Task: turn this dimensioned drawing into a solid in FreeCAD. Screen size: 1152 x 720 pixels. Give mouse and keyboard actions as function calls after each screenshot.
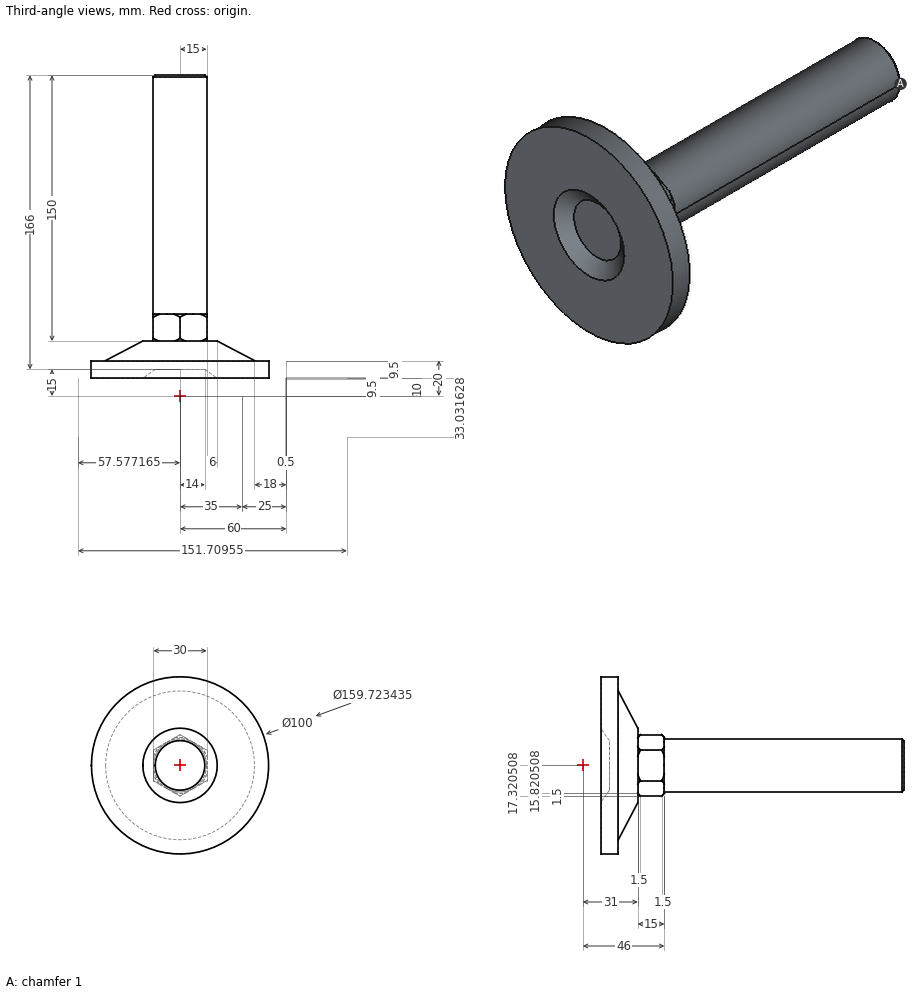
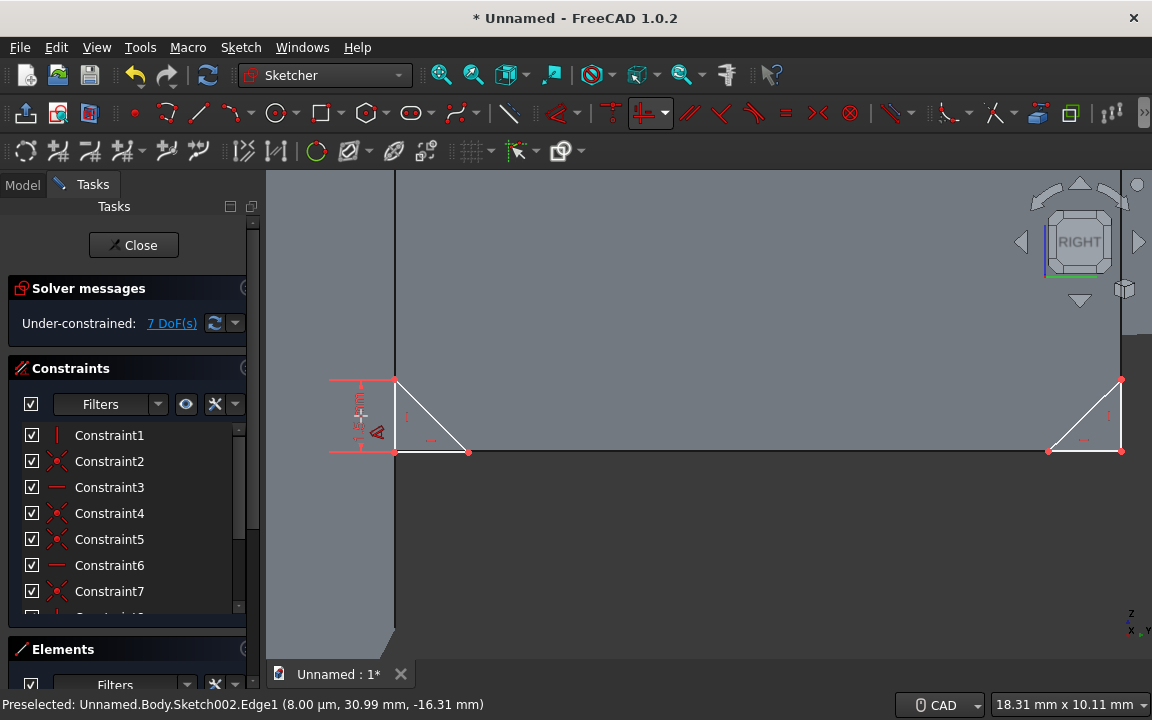
click(417, 452)
click(431, 486)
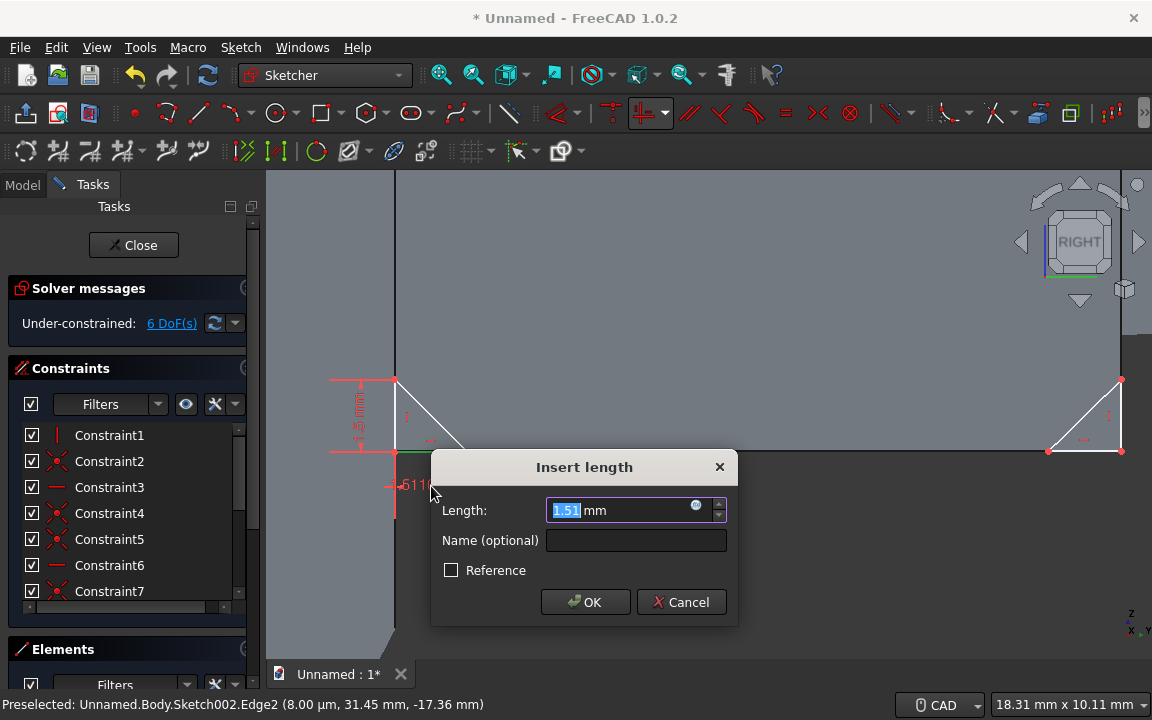
text(1.5)
key(Return)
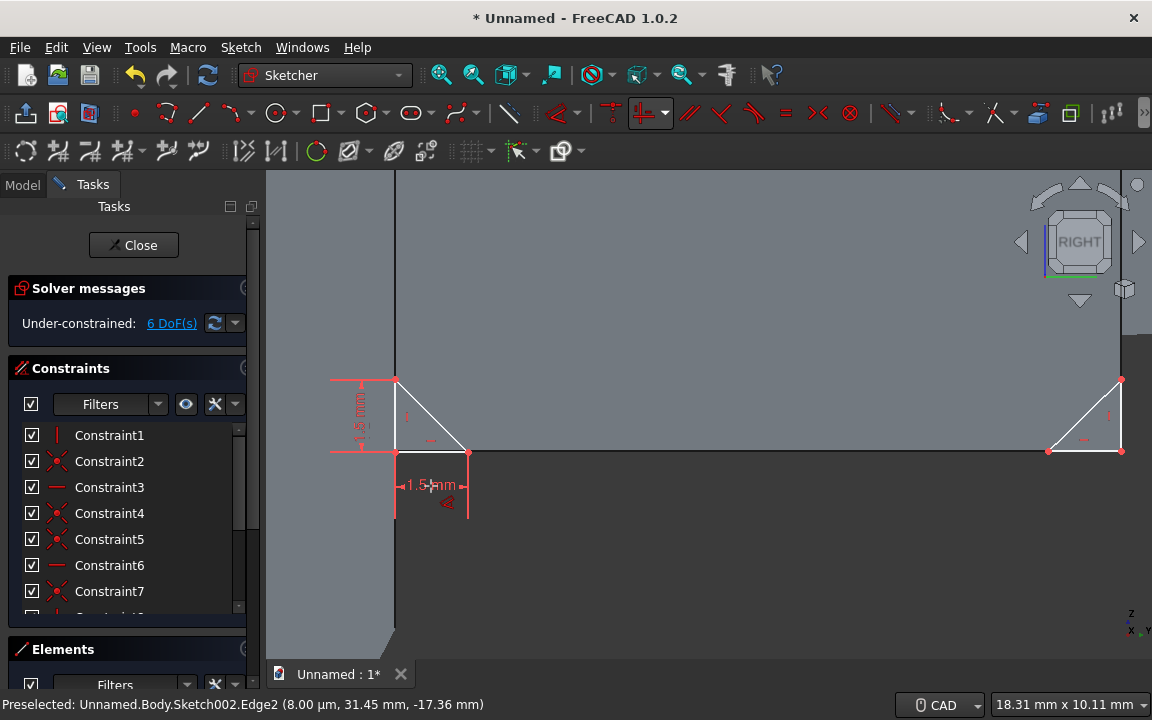
scroll(401, 415, down, 2)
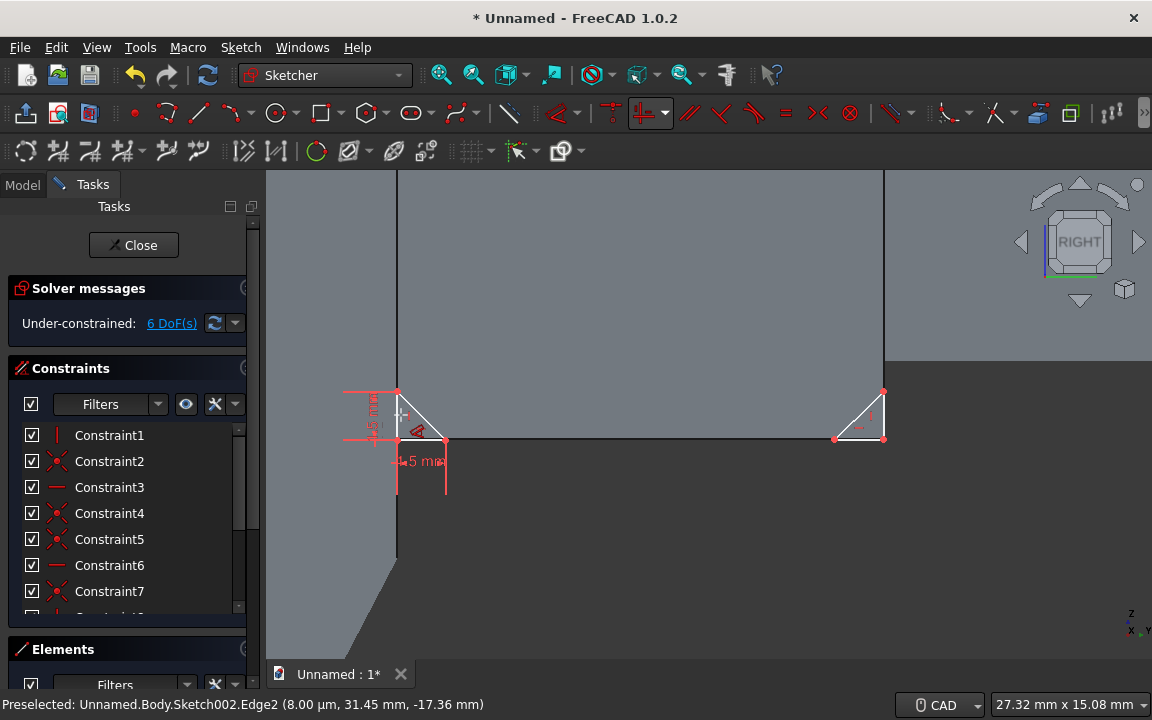
scroll(850, 440, up, 2)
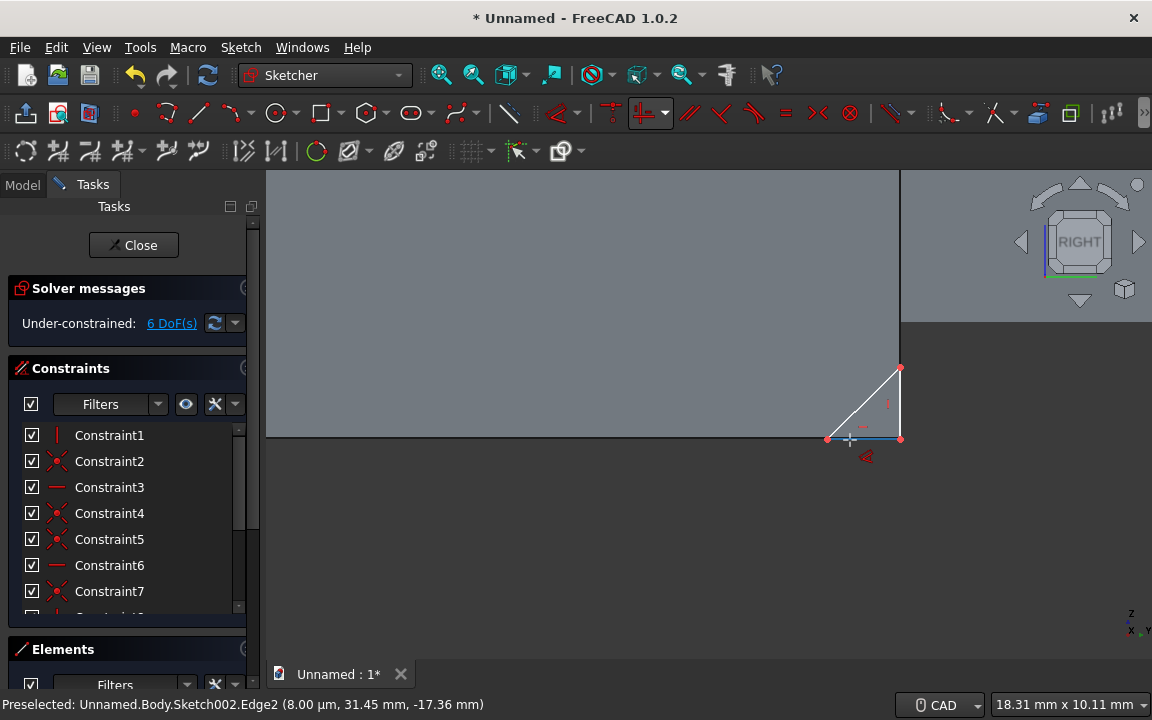
click(849, 439)
click(864, 473)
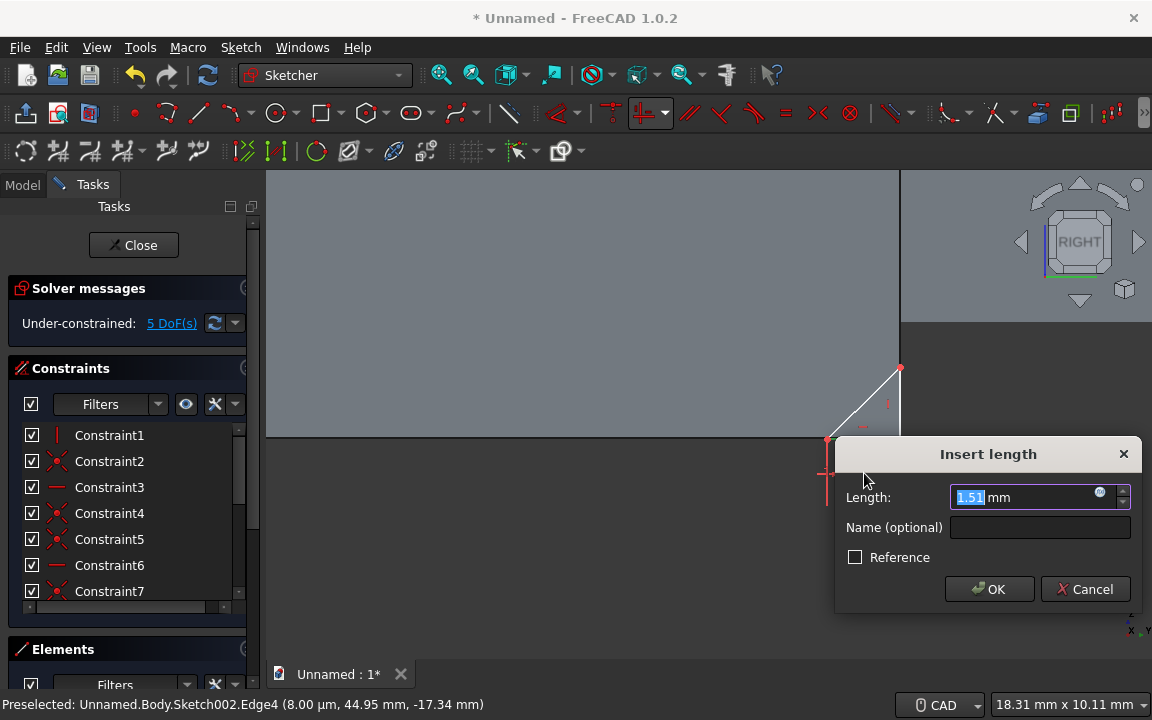
text(1.5)
key(Return)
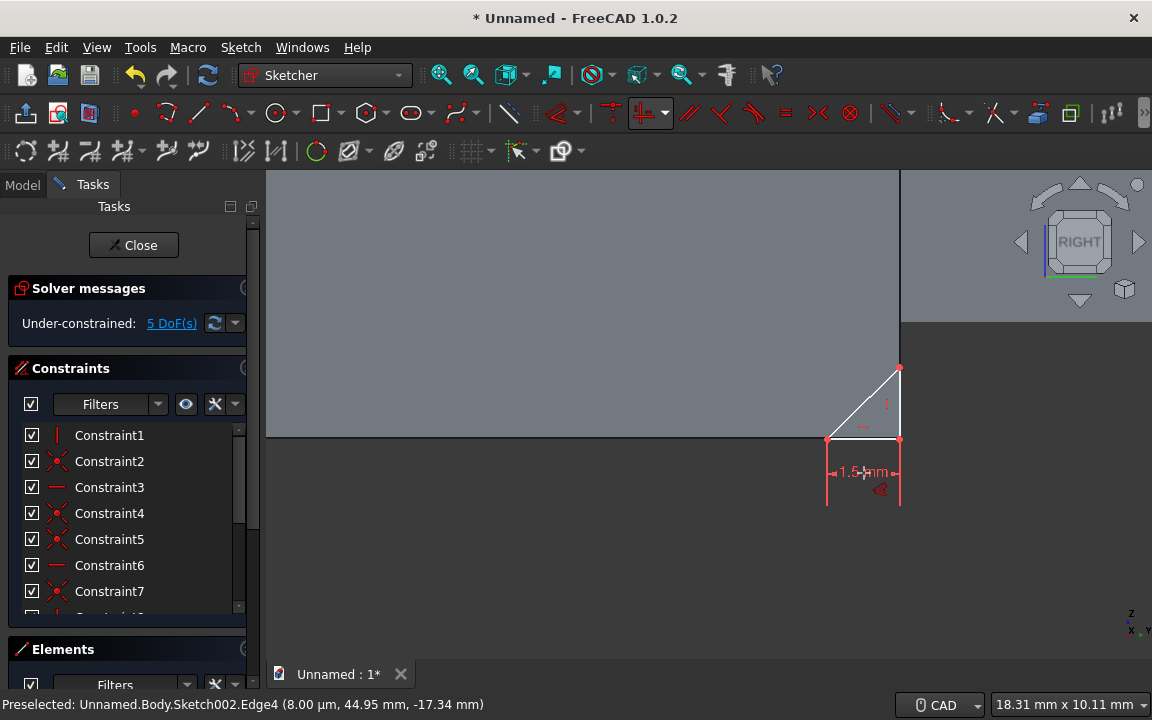
click(900, 418)
click(934, 403)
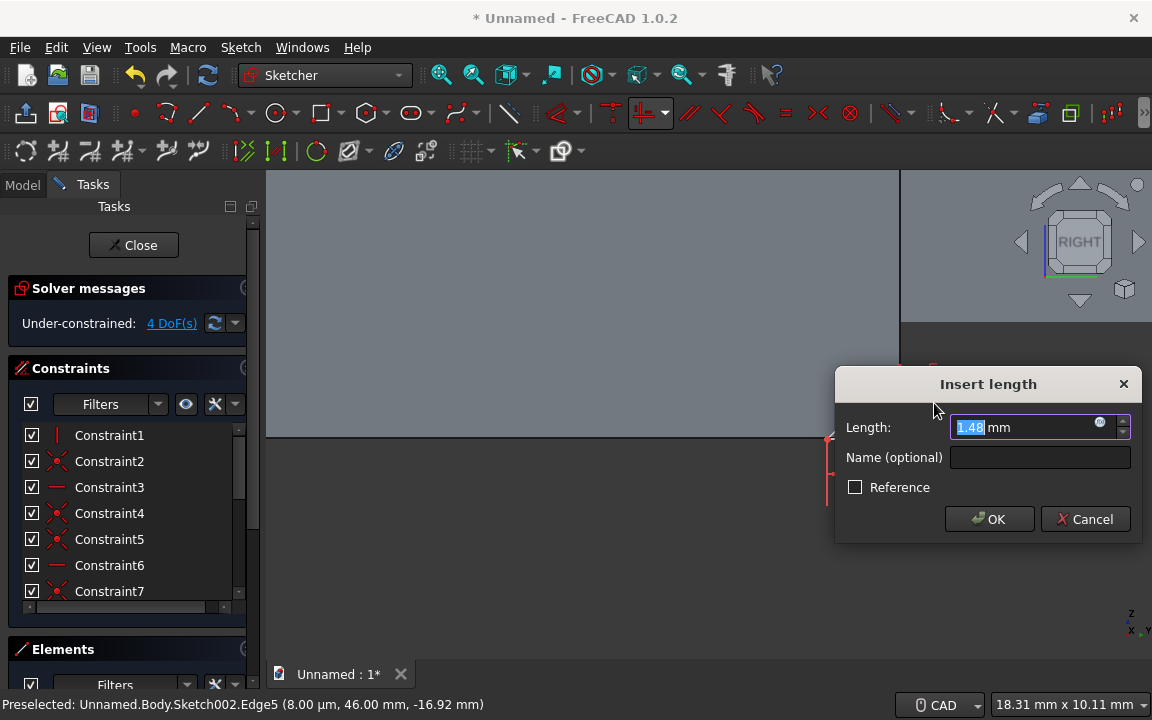
text(1.5)
key(Return)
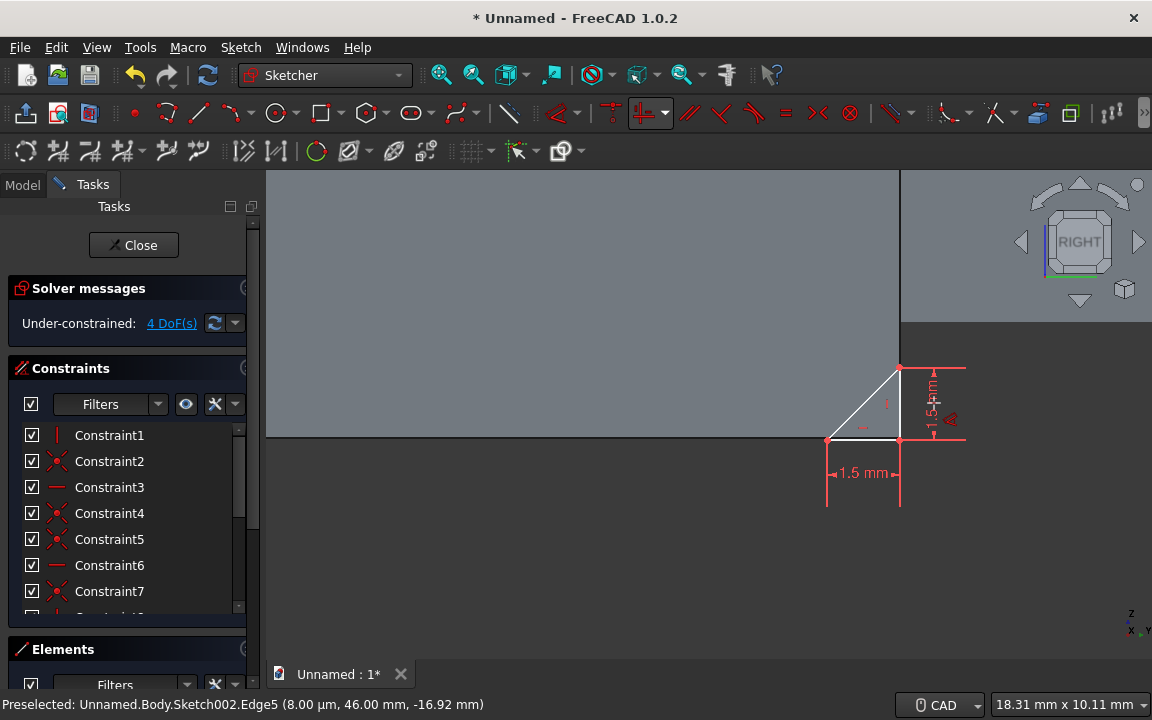
scroll(851, 440, down, 2)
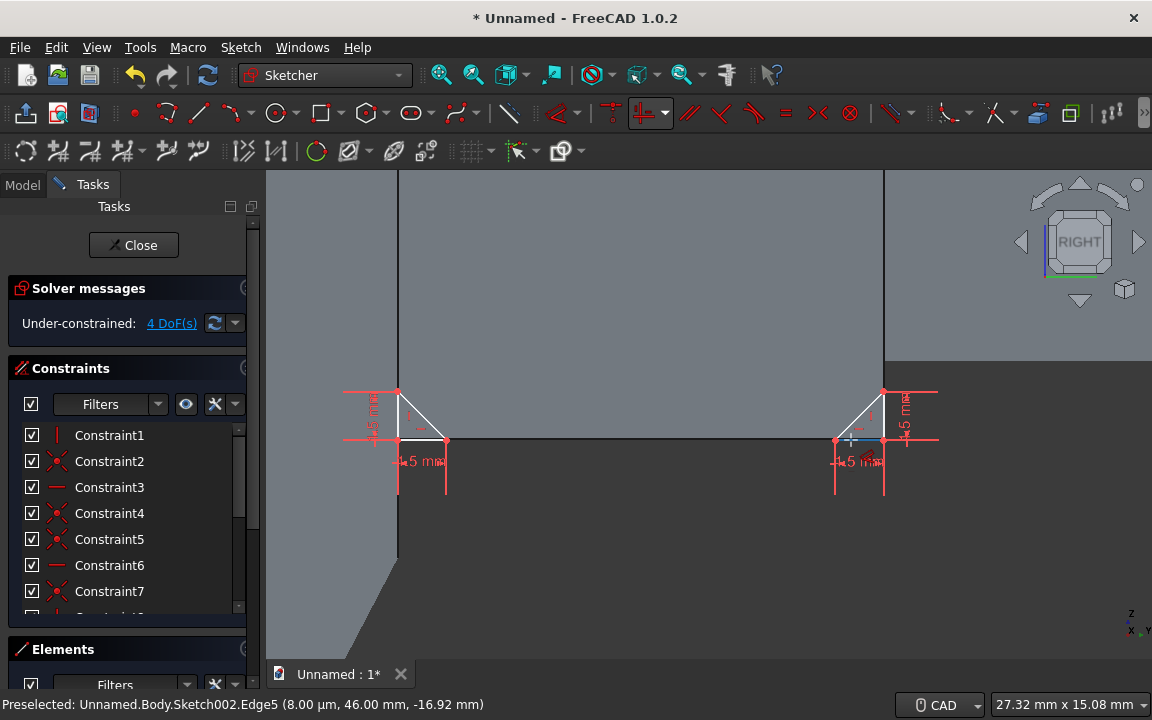
click(398, 392)
click(346, 450)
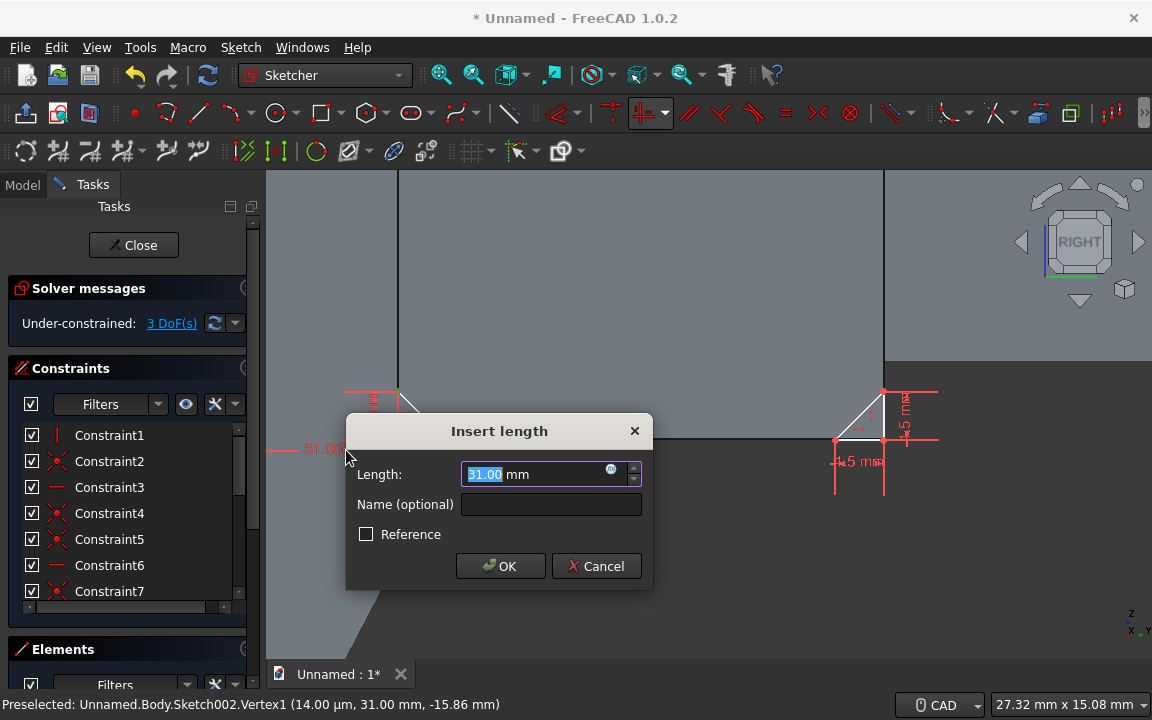
text(31)
key(Return)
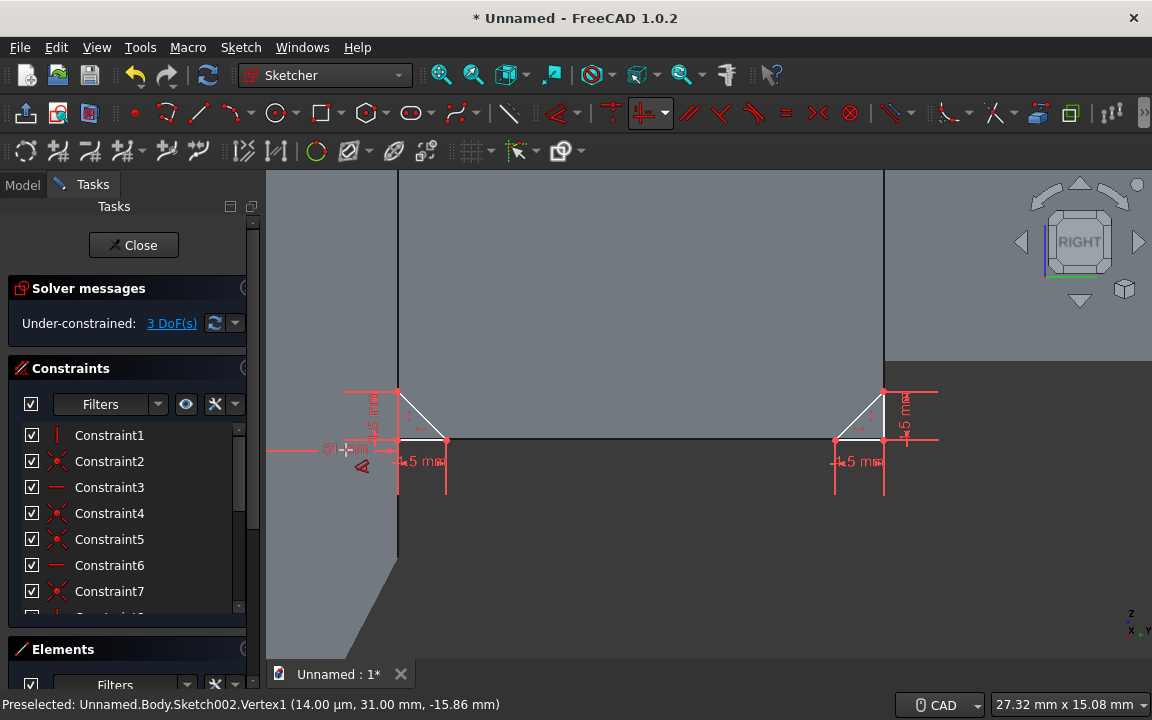
click(884, 440)
click(589, 474)